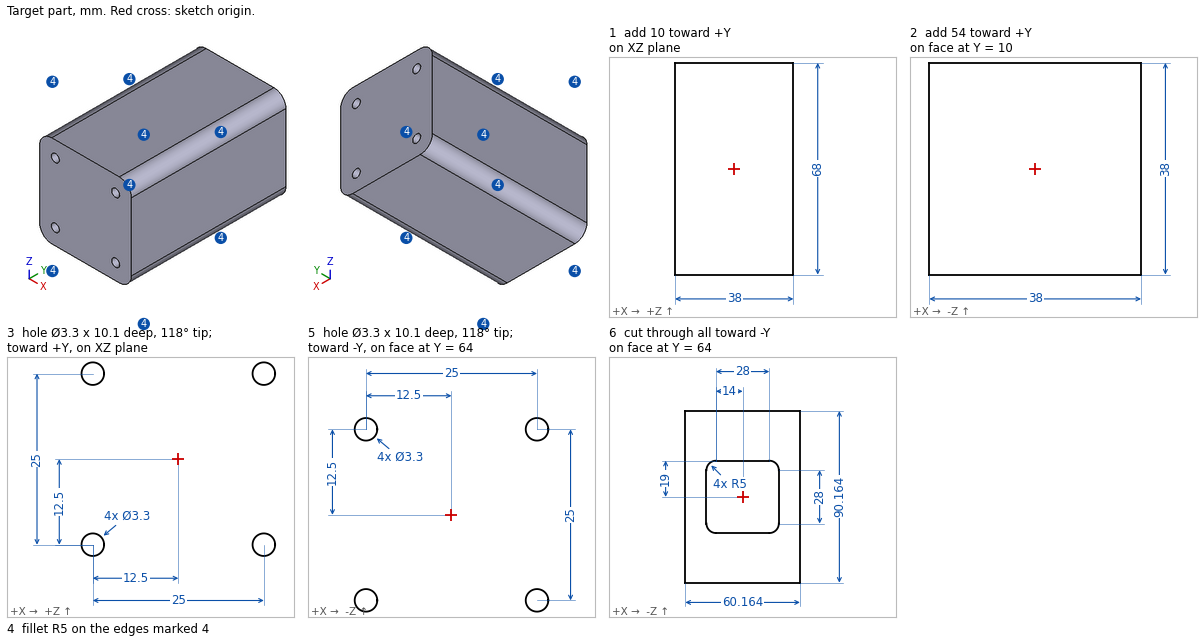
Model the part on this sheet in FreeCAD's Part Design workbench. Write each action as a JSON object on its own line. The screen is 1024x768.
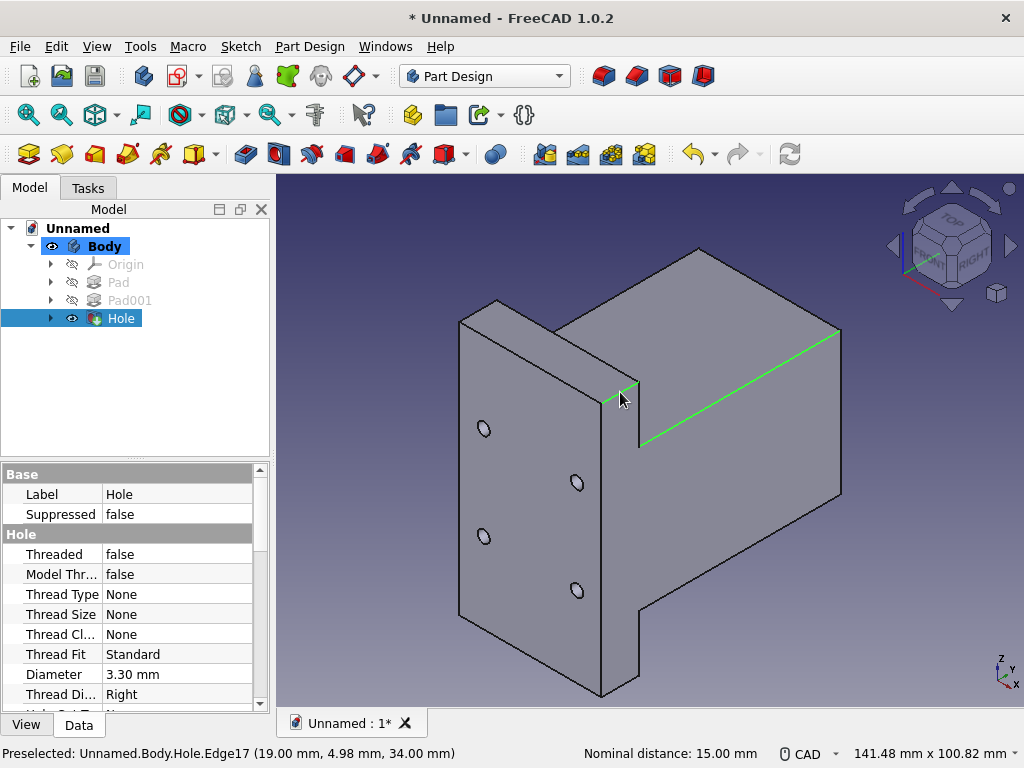
{"action": "key", "text": "2"}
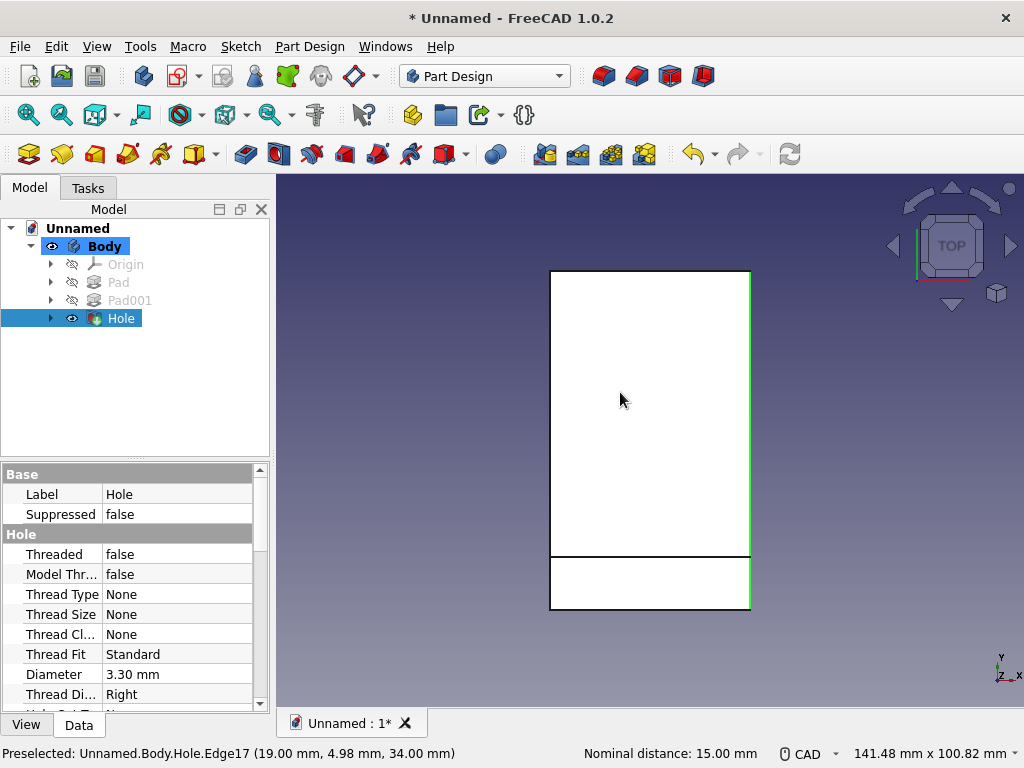
{"action": "left_click", "coordinate": [550, 413], "text": "ctrl"}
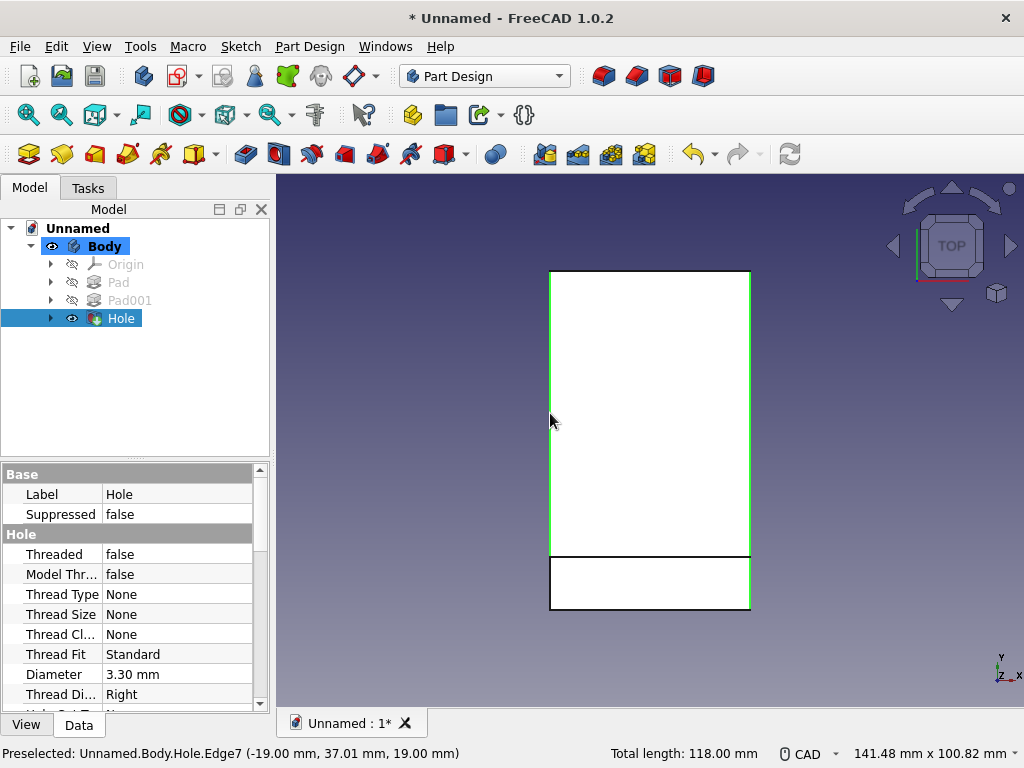
{"action": "left_click", "coordinate": [550, 582], "text": "ctrl"}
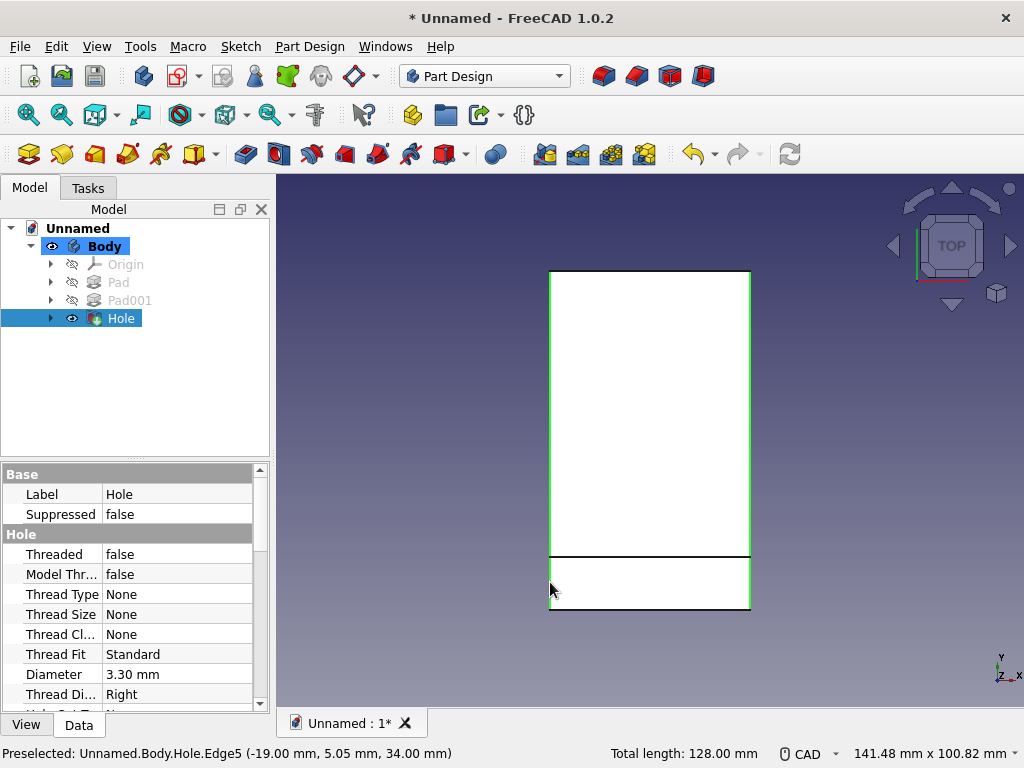
{"action": "key", "text": "1"}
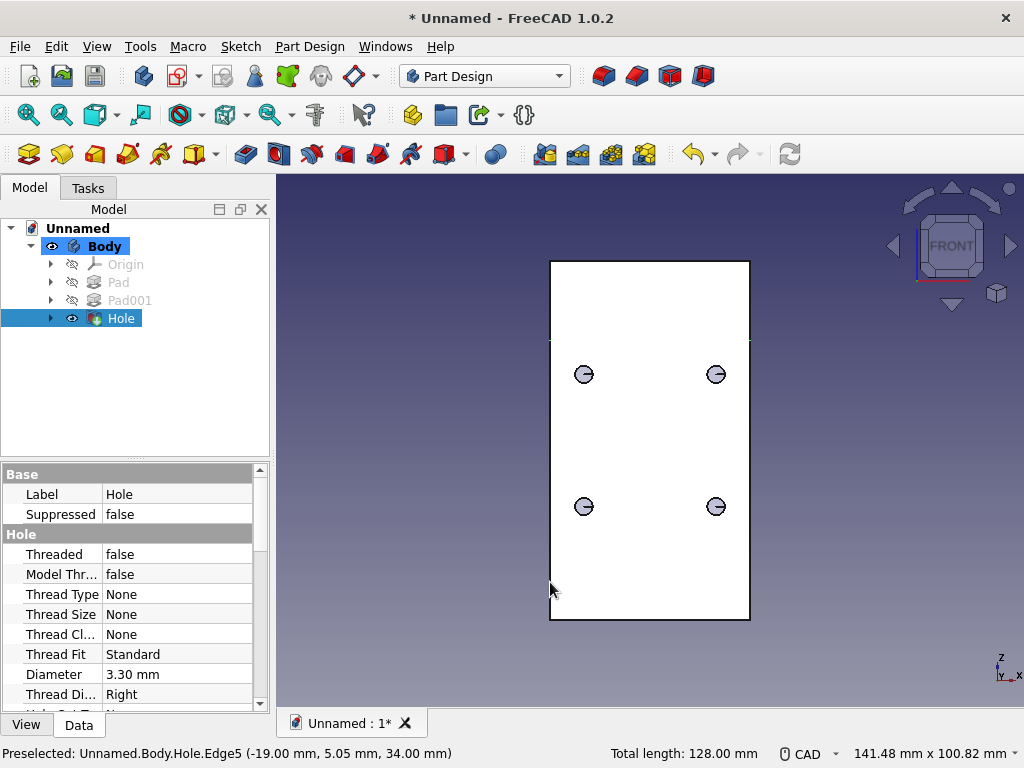
{"action": "key", "text": "3"}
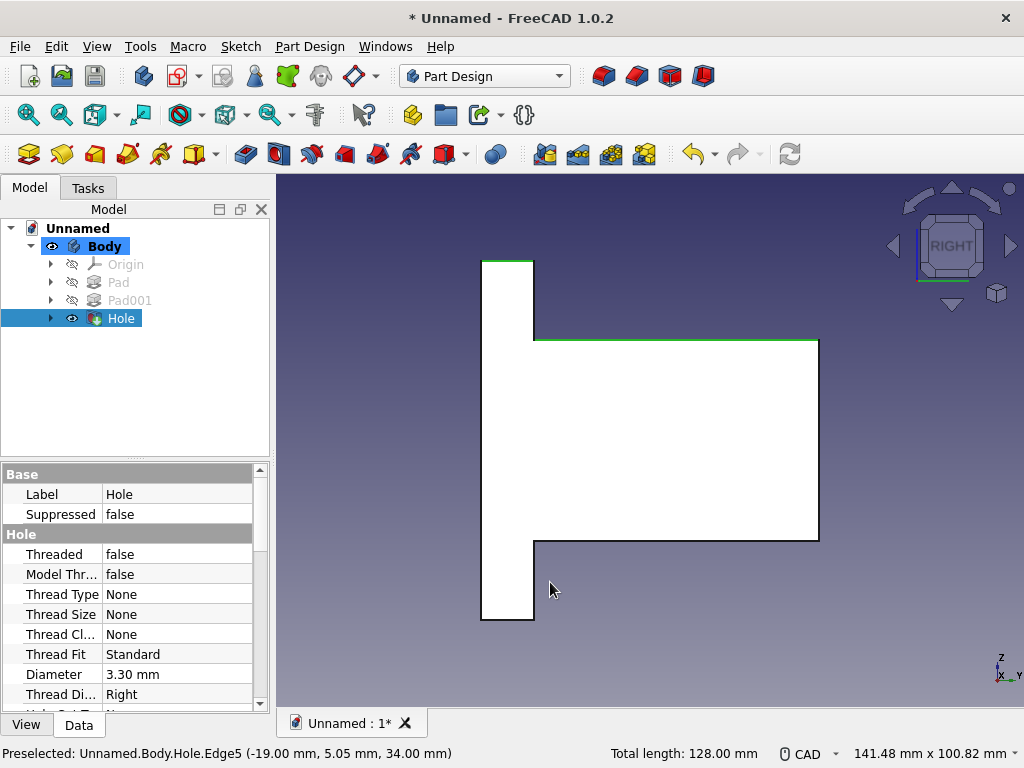
{"action": "left_click", "coordinate": [676, 540], "text": "ctrl"}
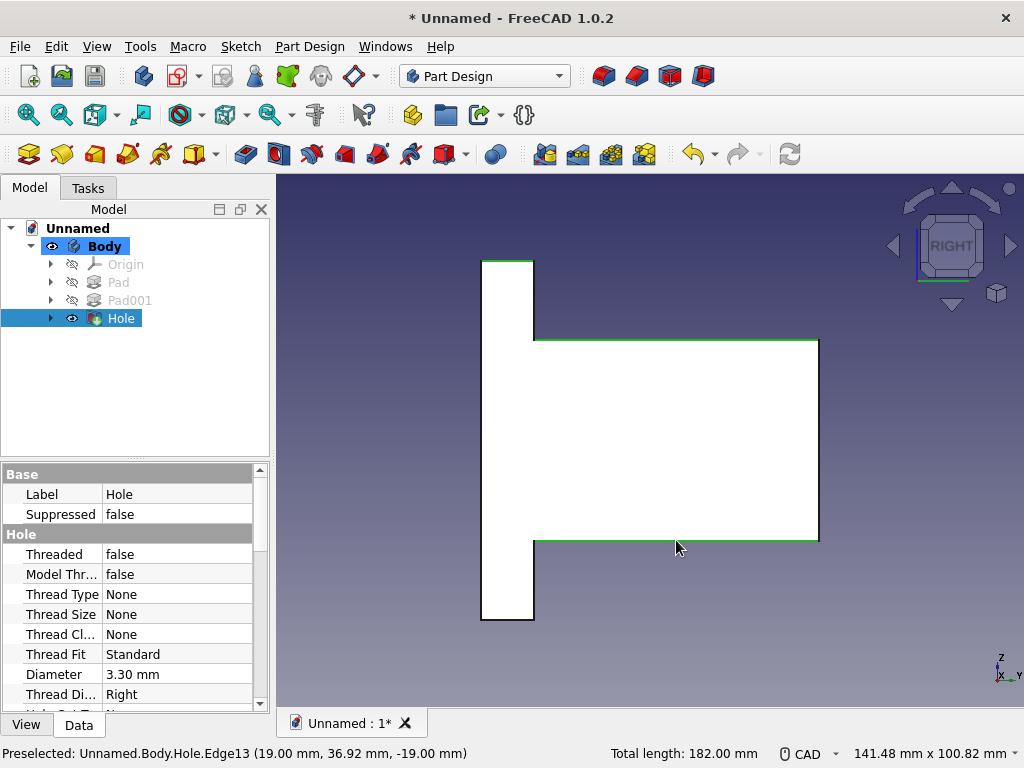
{"action": "left_click", "coordinate": [507, 619], "text": "ctrl"}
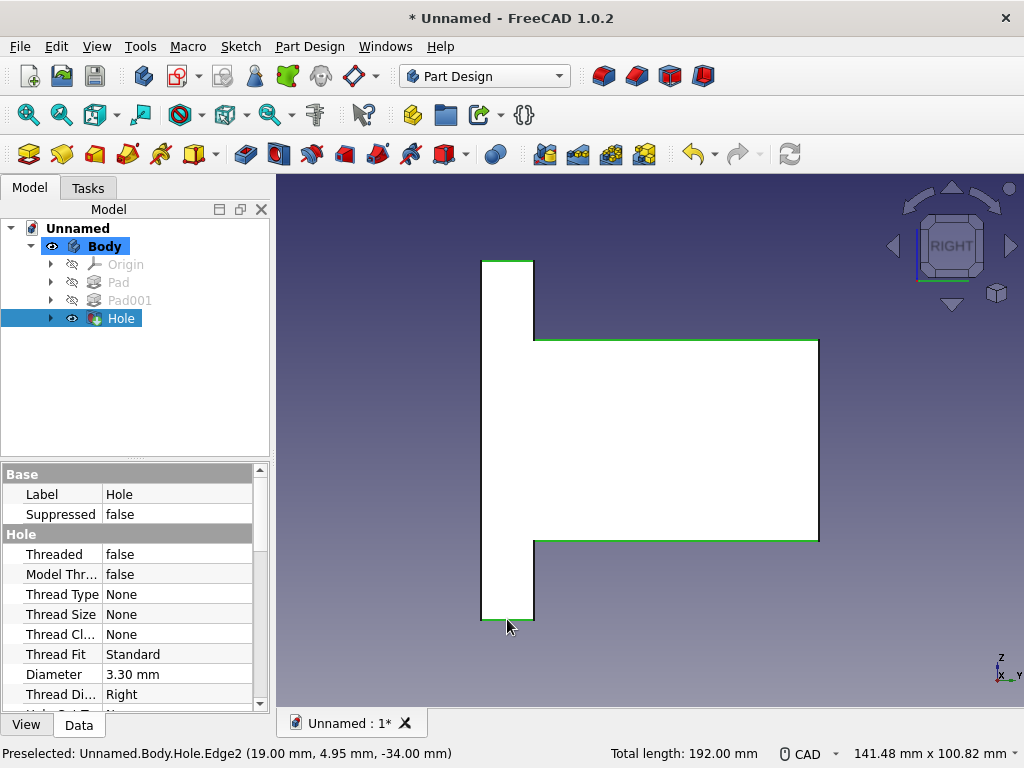
{"action": "key", "text": "5"}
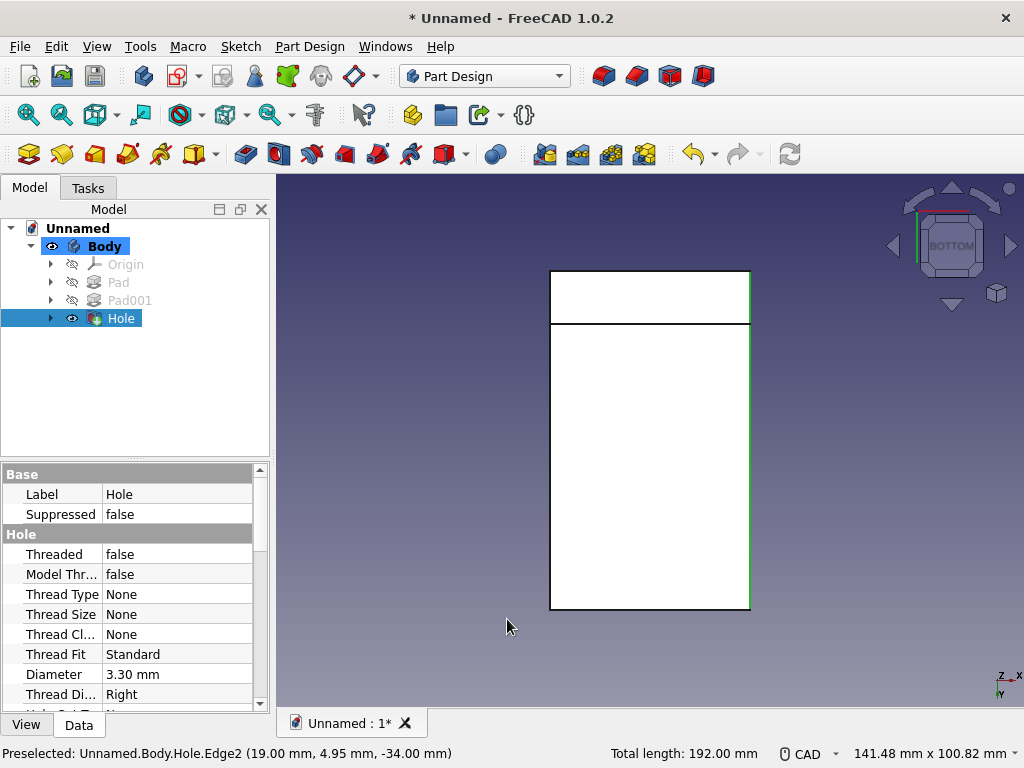
{"action": "left_click", "coordinate": [550, 466], "text": "ctrl"}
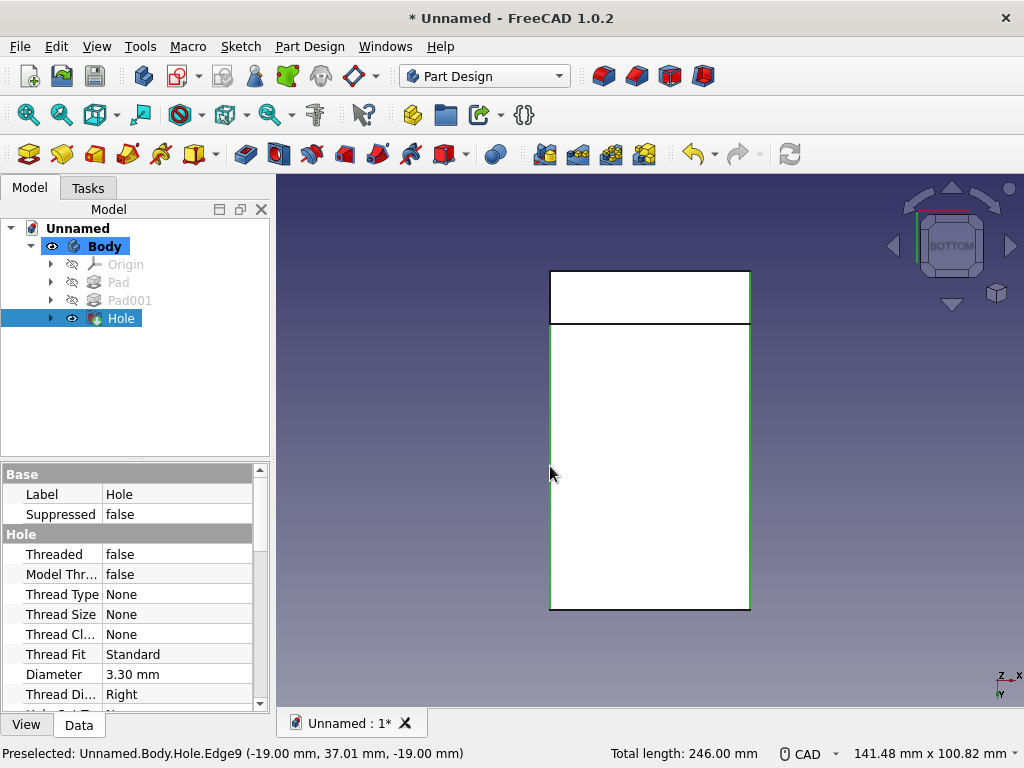
{"action": "left_click", "coordinate": [550, 297], "text": "ctrl"}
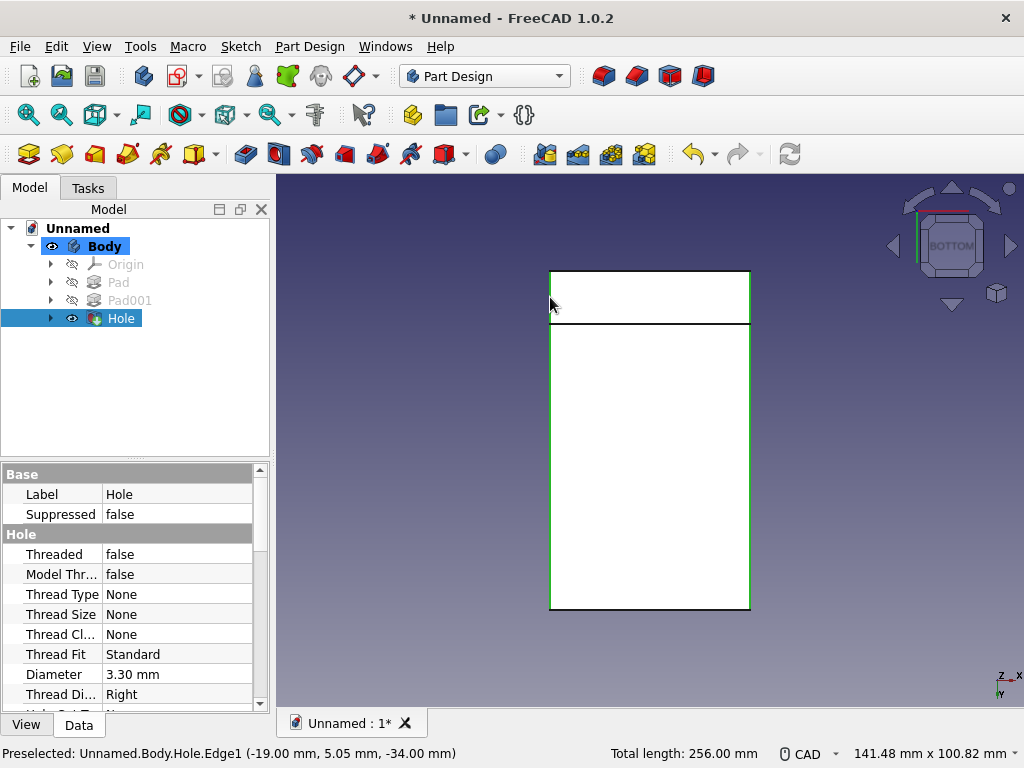
{"action": "left_click", "coordinate": [604, 76]}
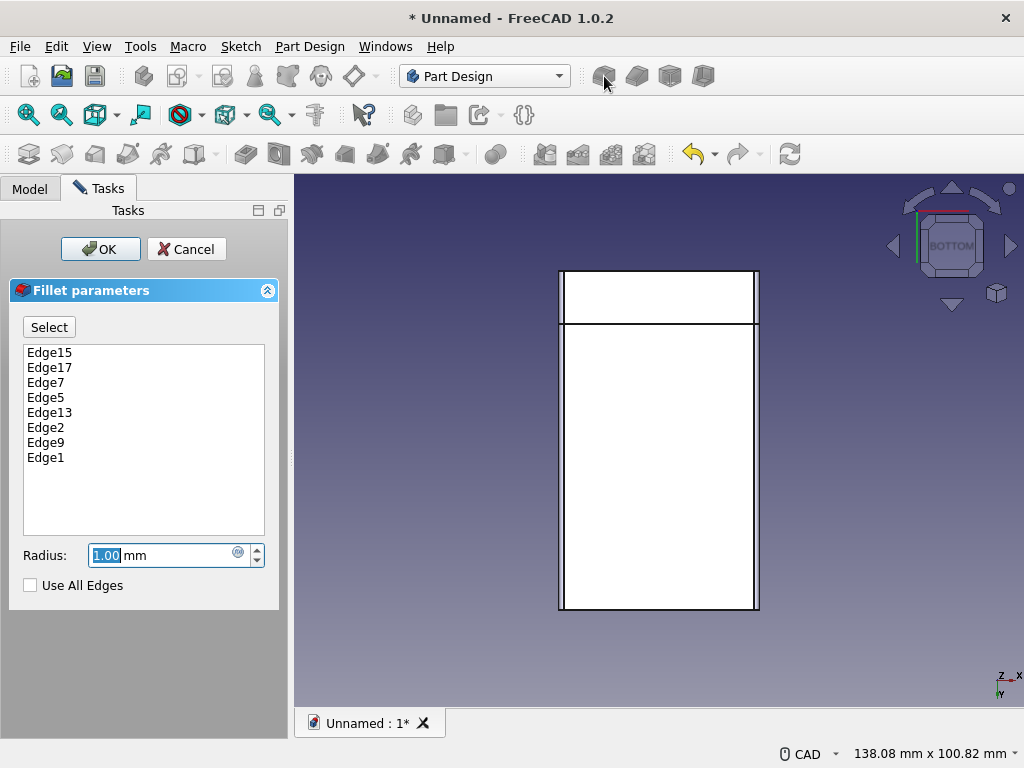
{"action": "type", "text": "5"}
{"action": "key", "text": "Tab"}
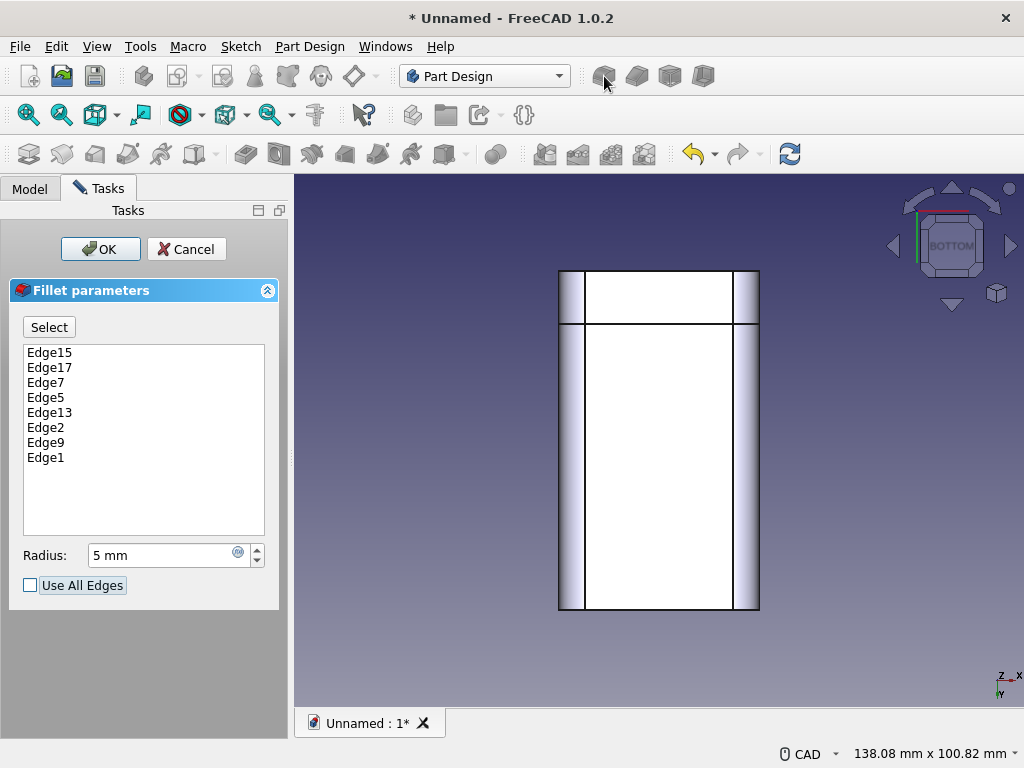
{"action": "left_click", "coordinate": [101, 249]}